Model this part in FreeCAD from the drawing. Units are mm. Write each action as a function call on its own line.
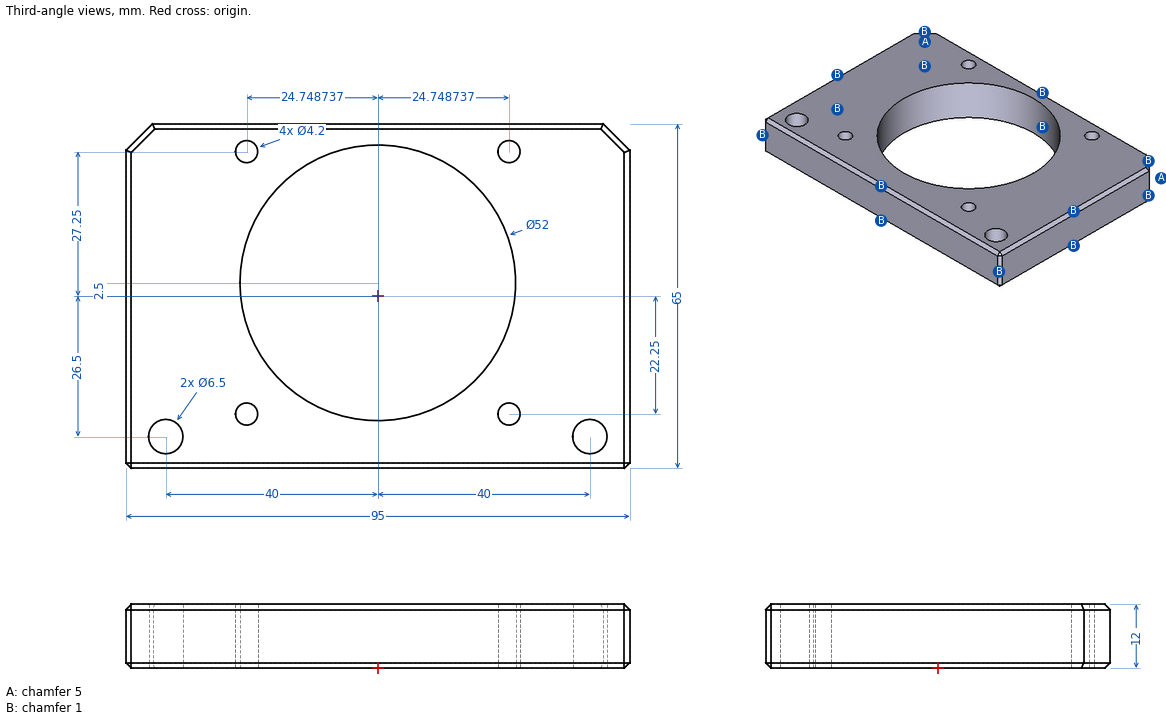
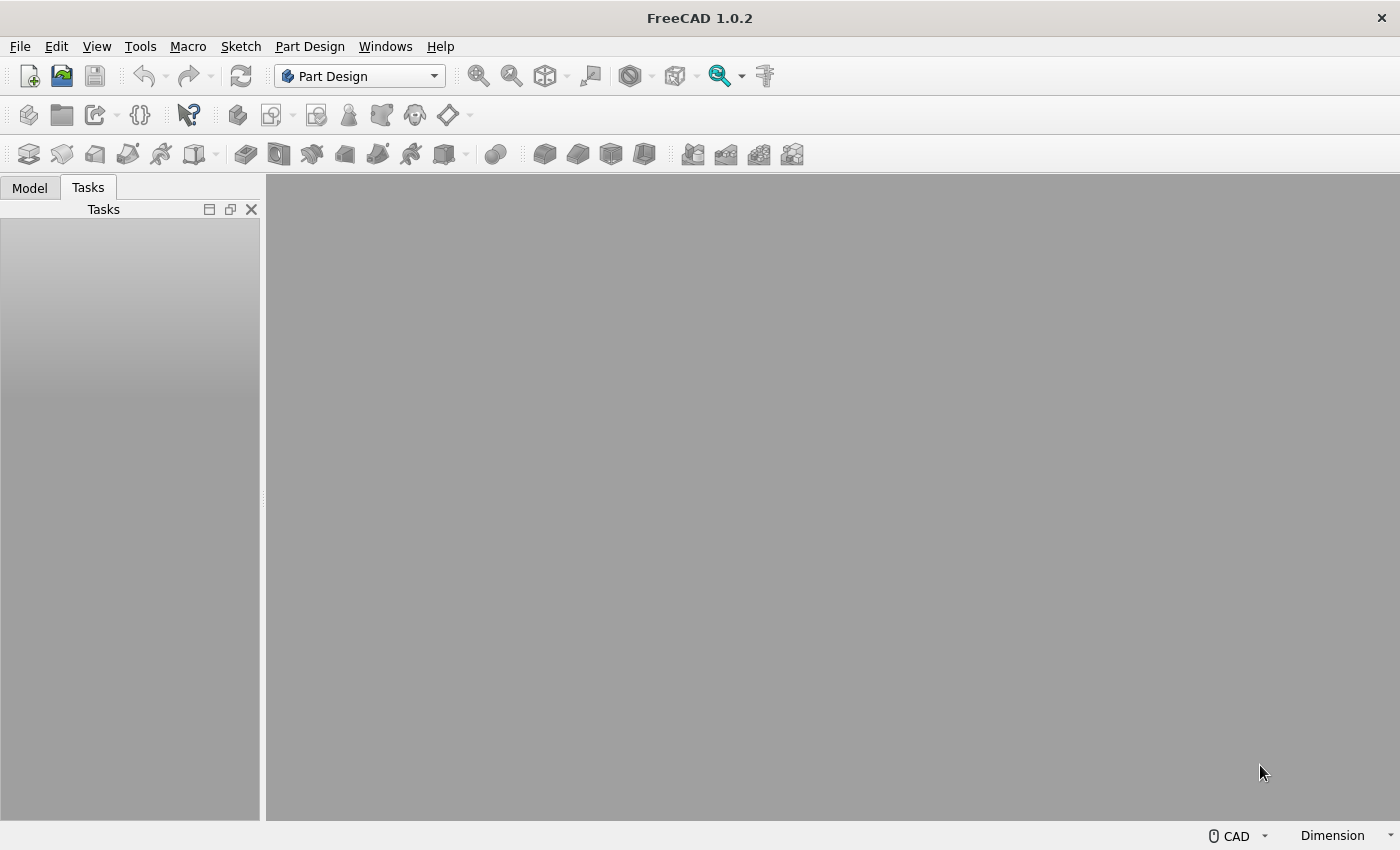
click(29, 76)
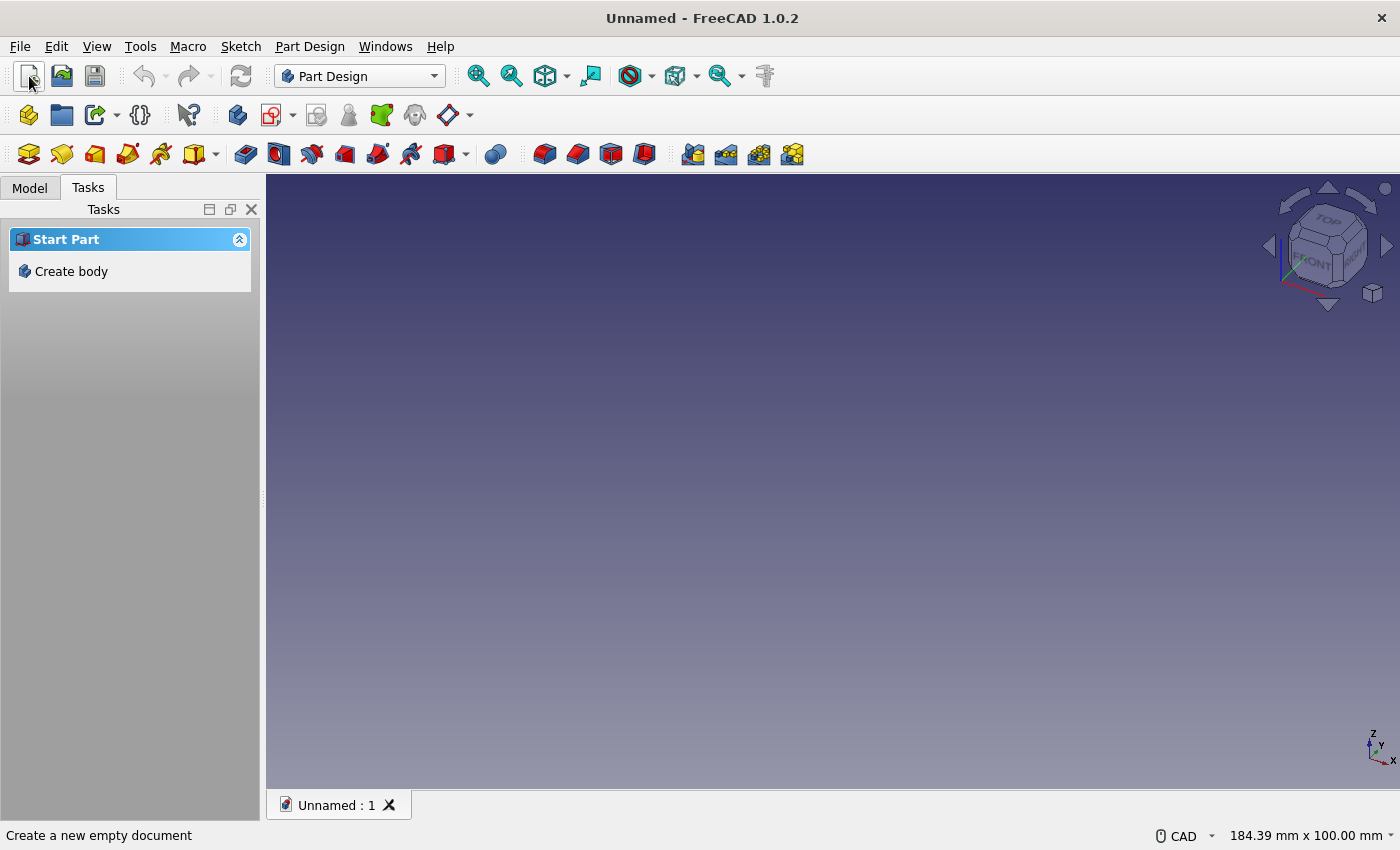
click(270, 116)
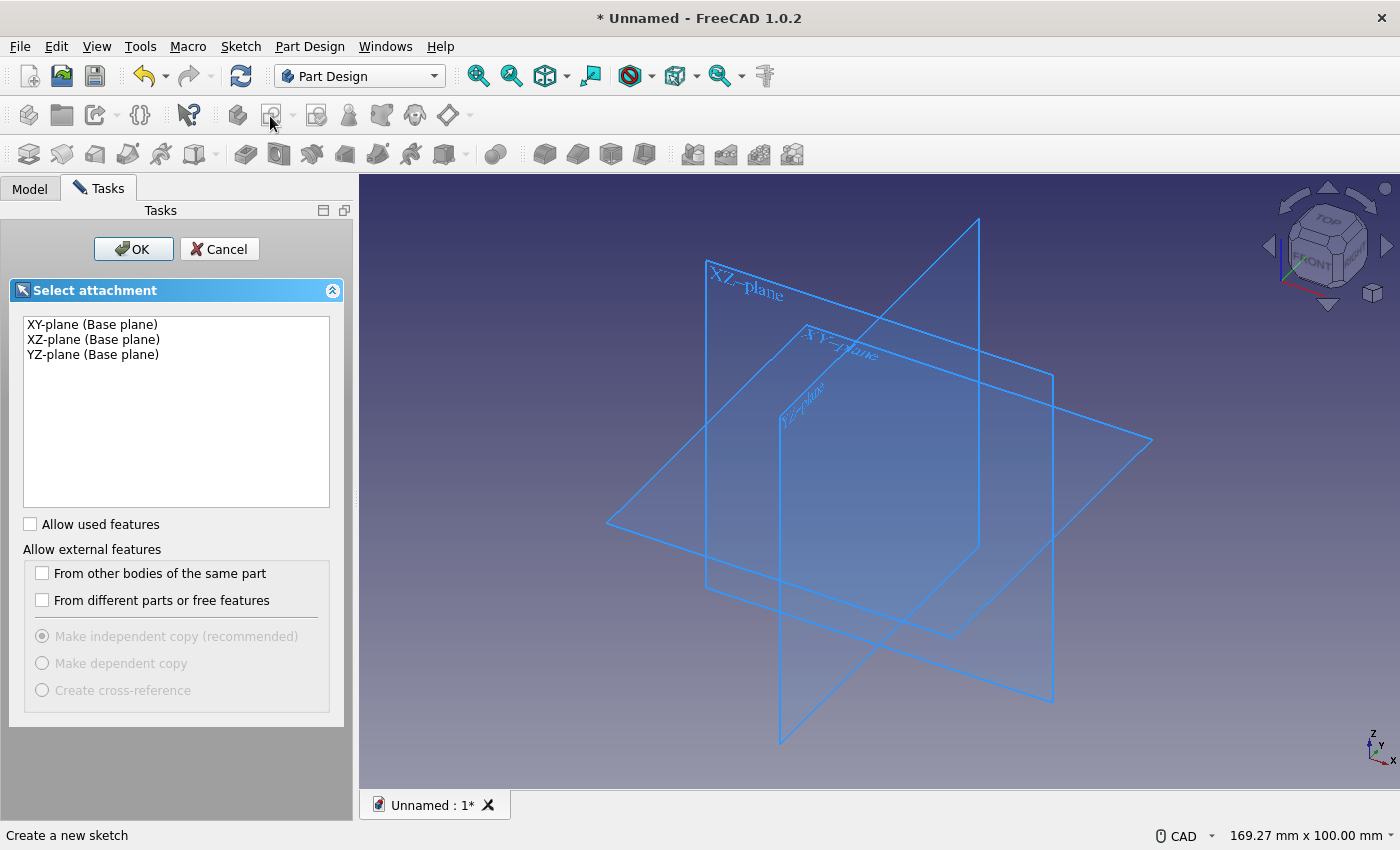
click(84, 324)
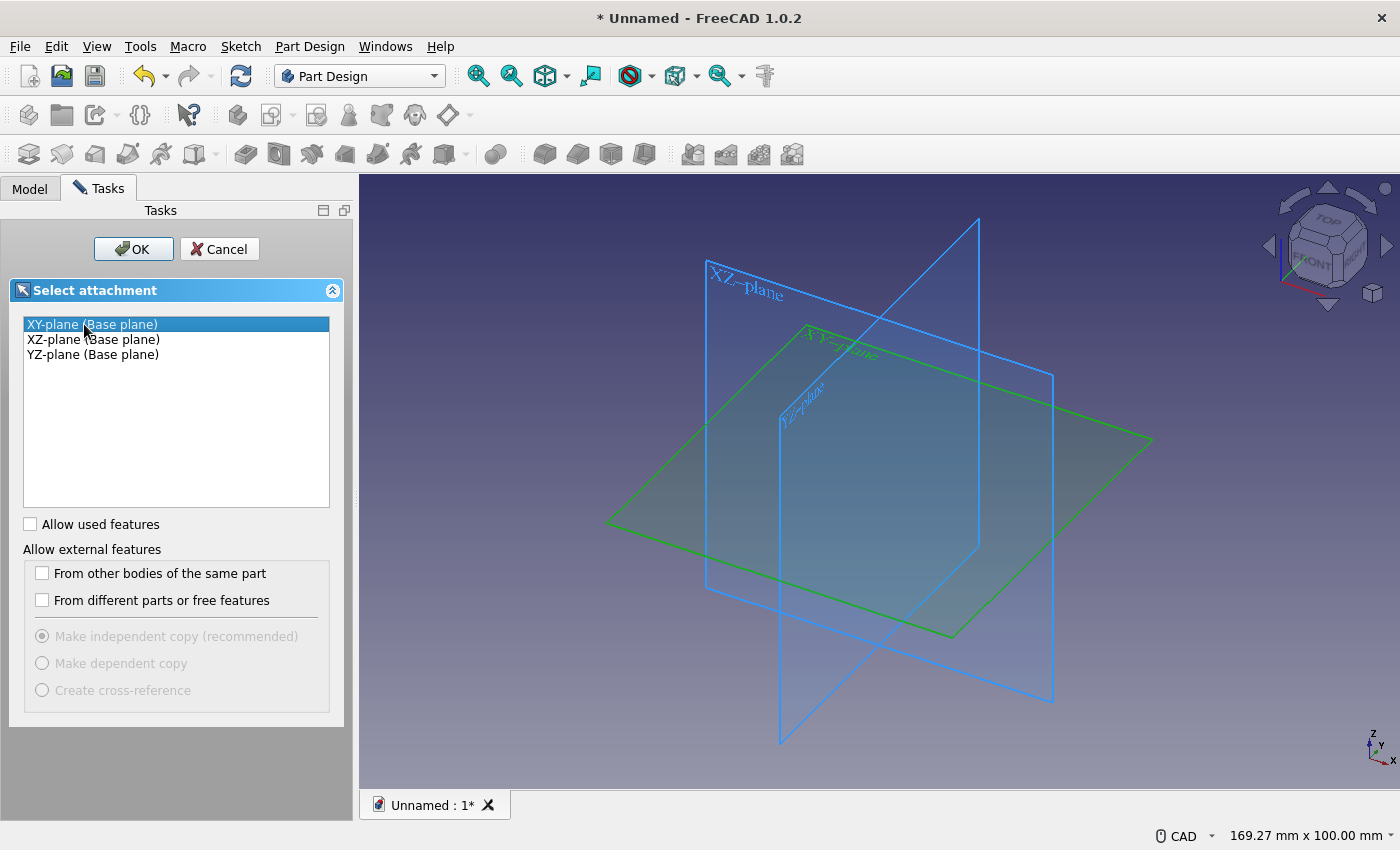
click(134, 249)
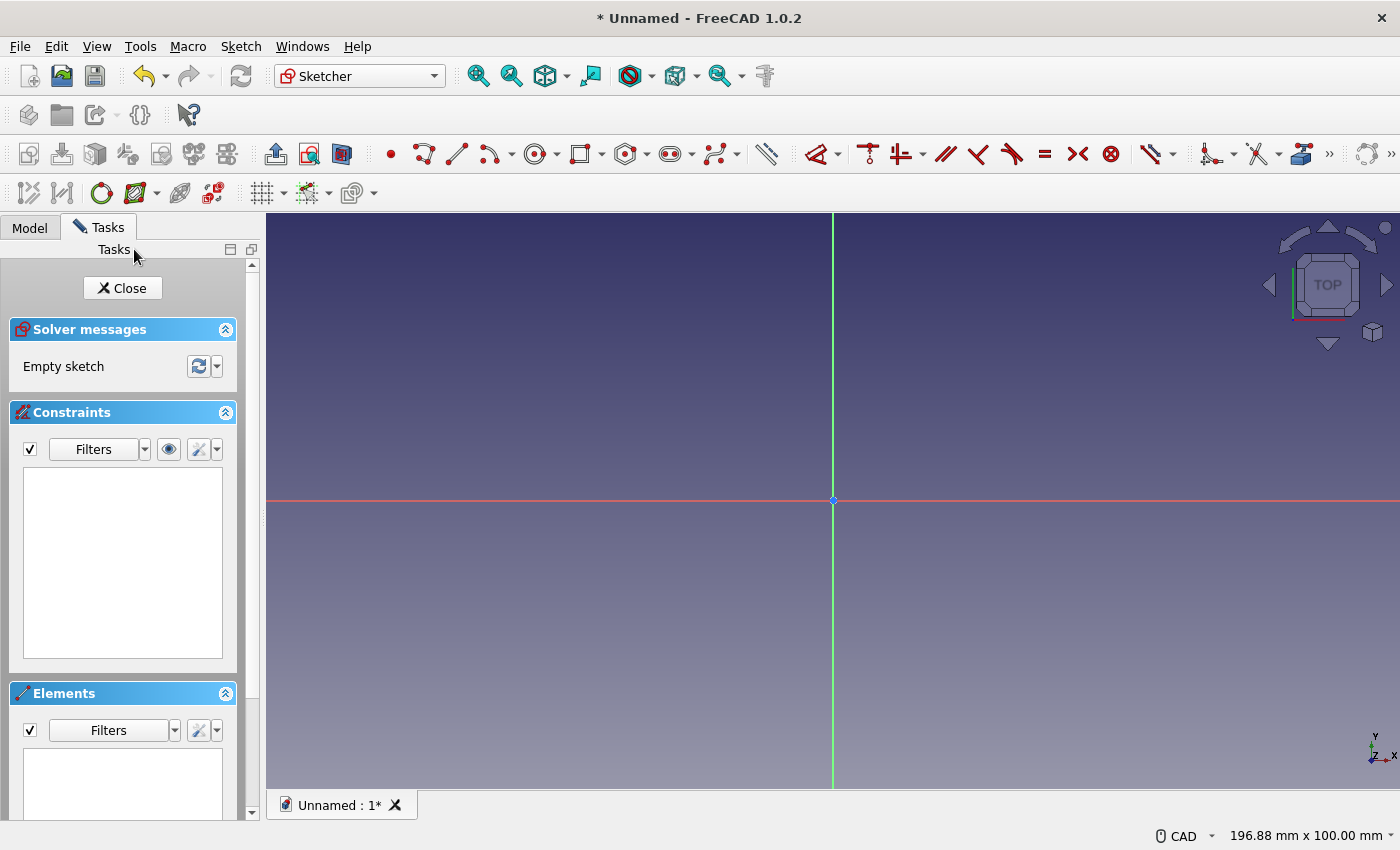
click(602, 154)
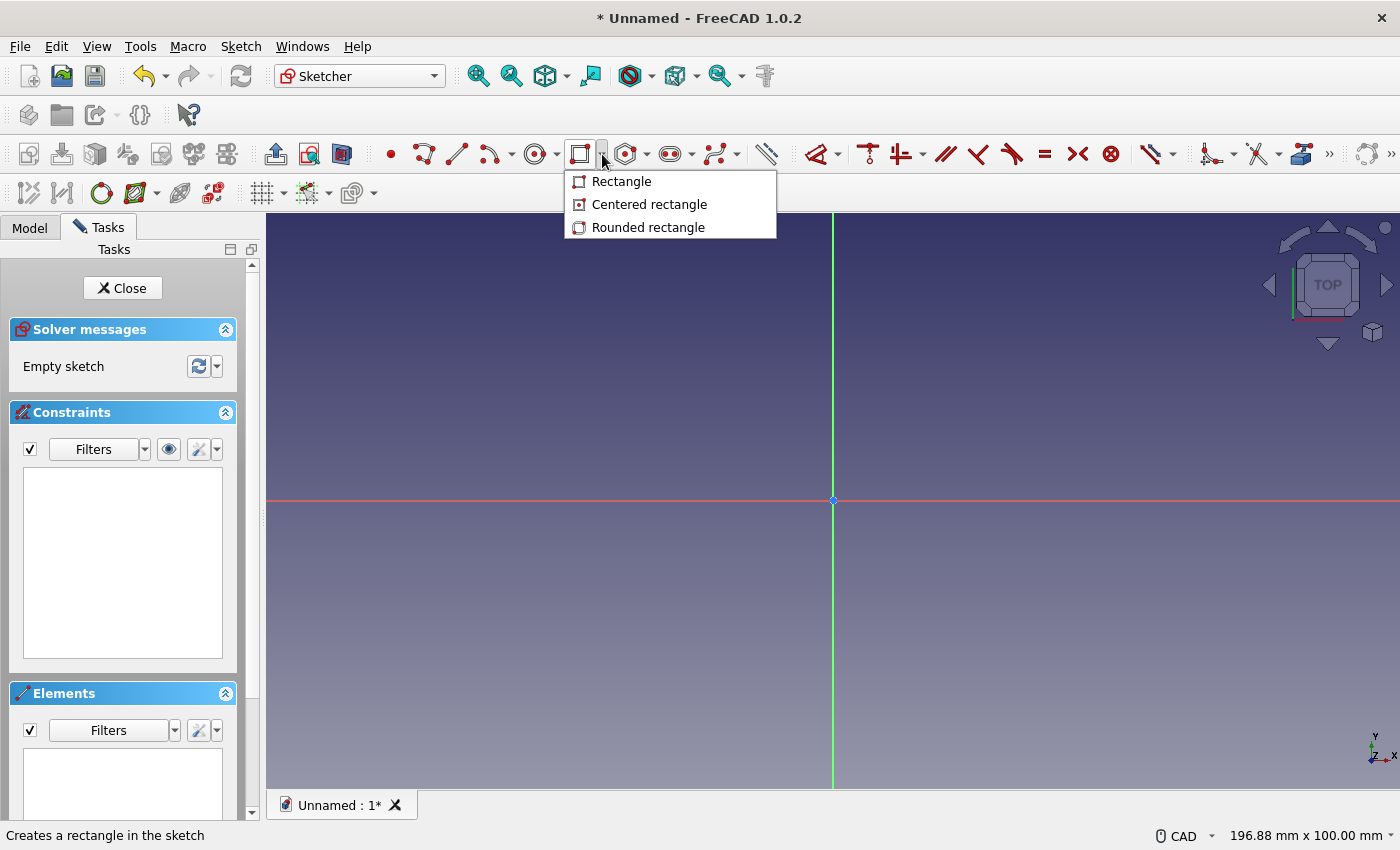
click(670, 204)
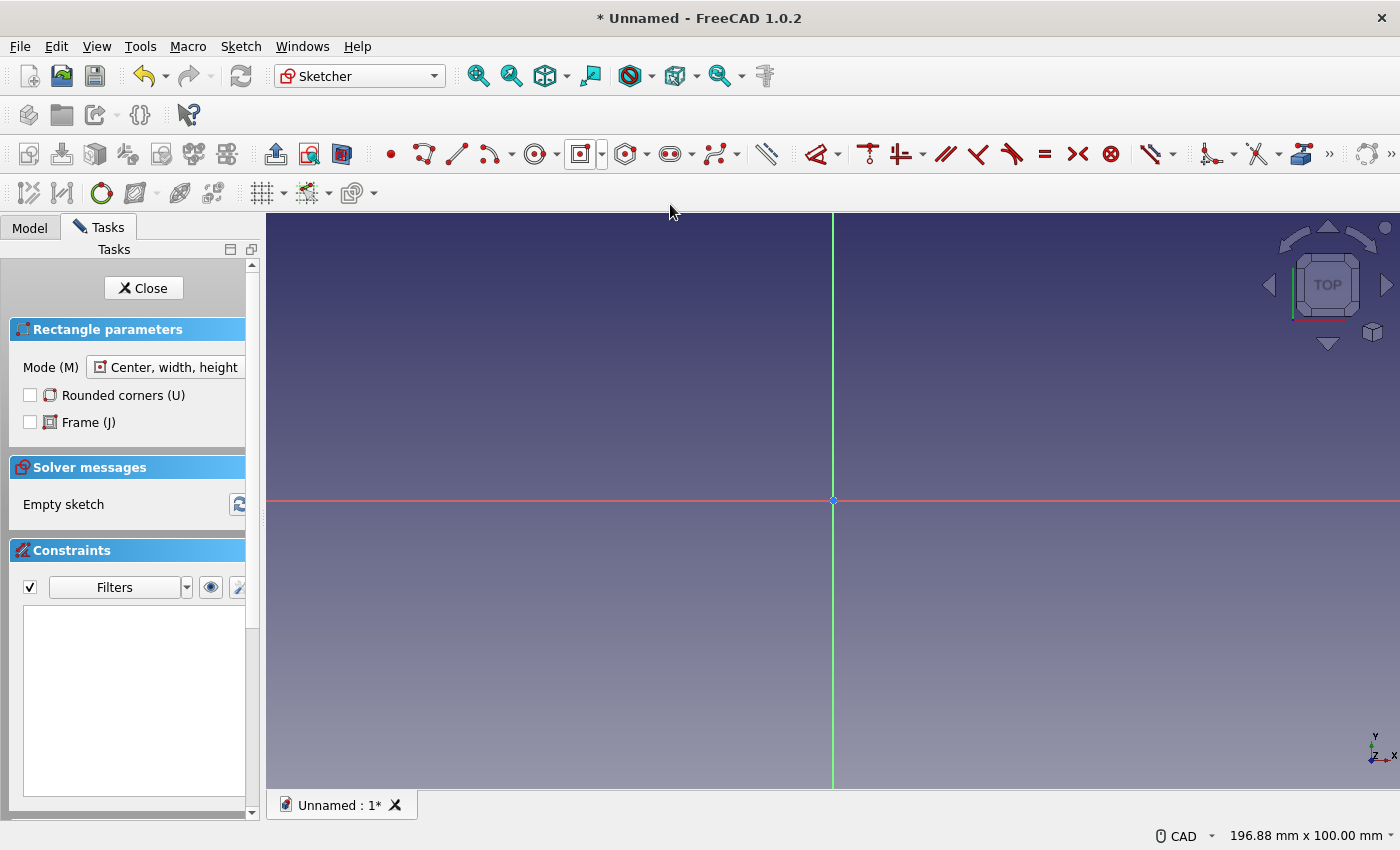
click(833, 501)
click(1107, 314)
key(Escape)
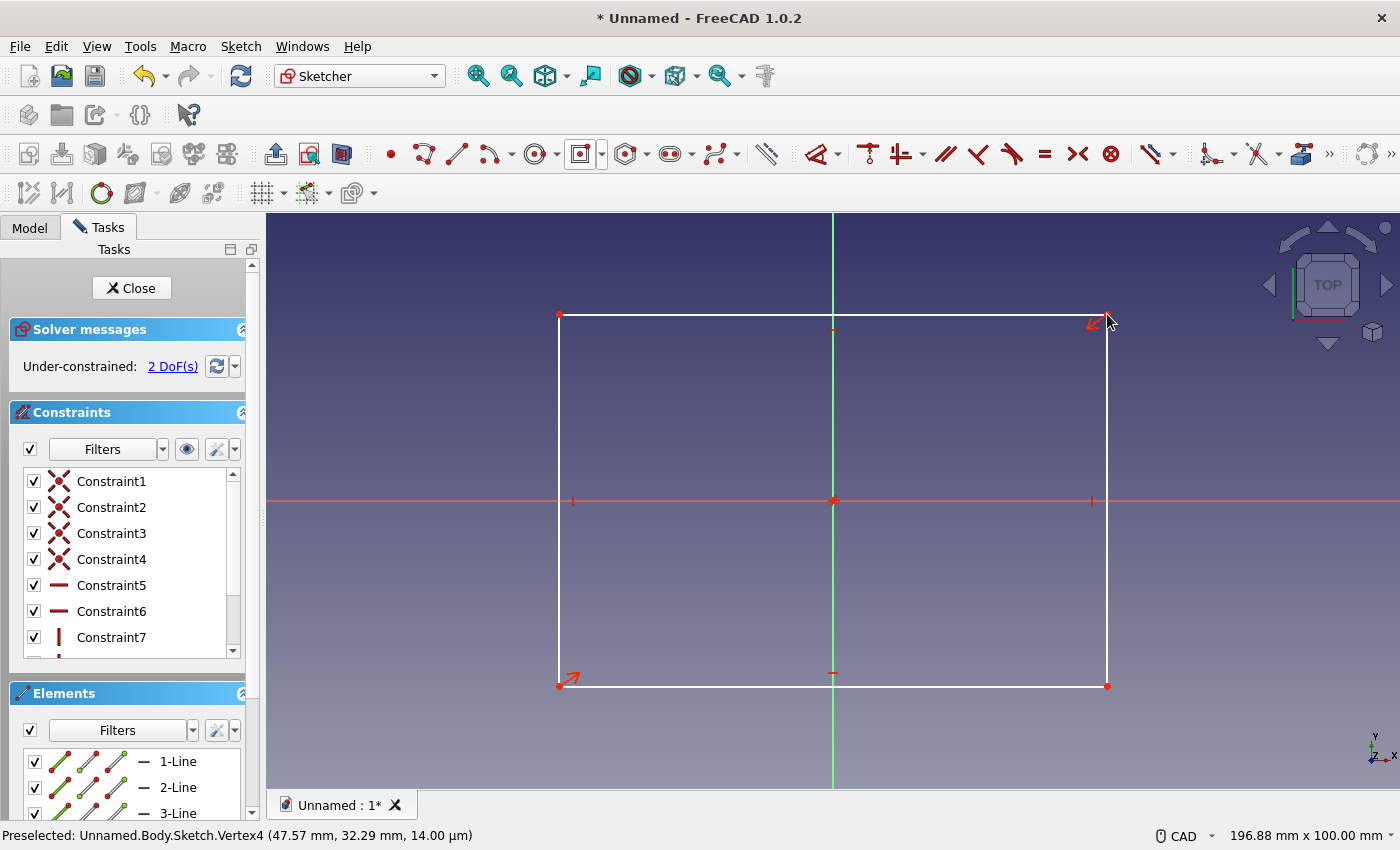
click(816, 154)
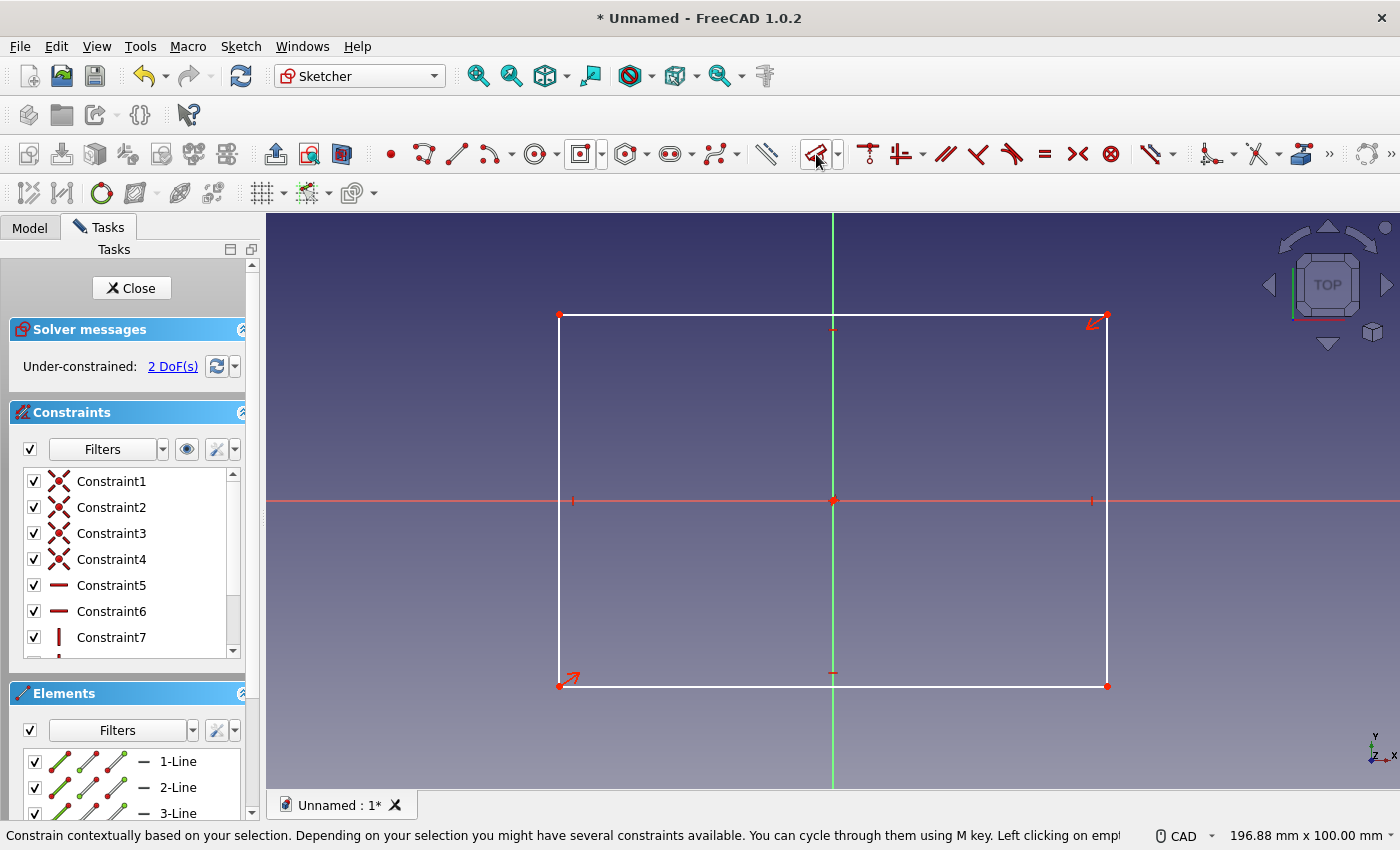
click(723, 687)
click(707, 721)